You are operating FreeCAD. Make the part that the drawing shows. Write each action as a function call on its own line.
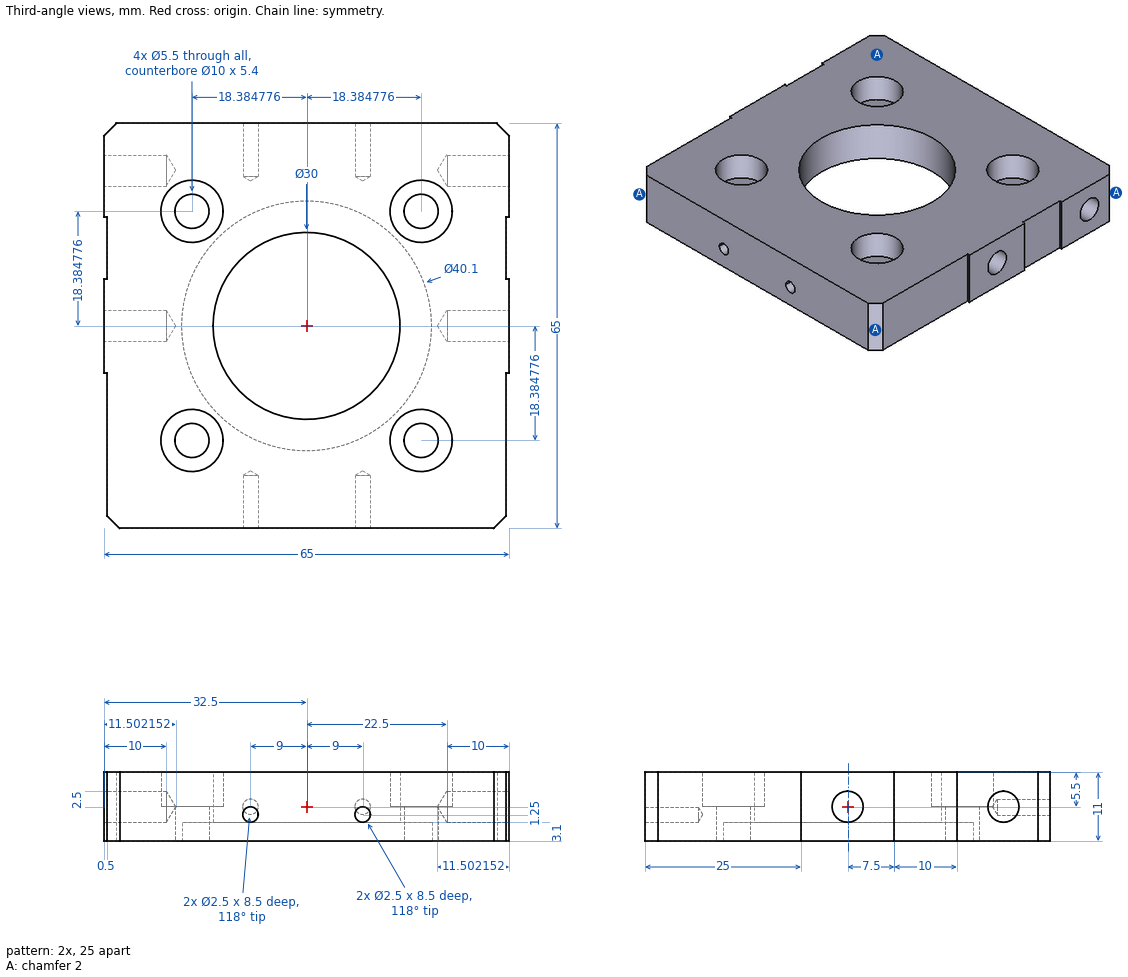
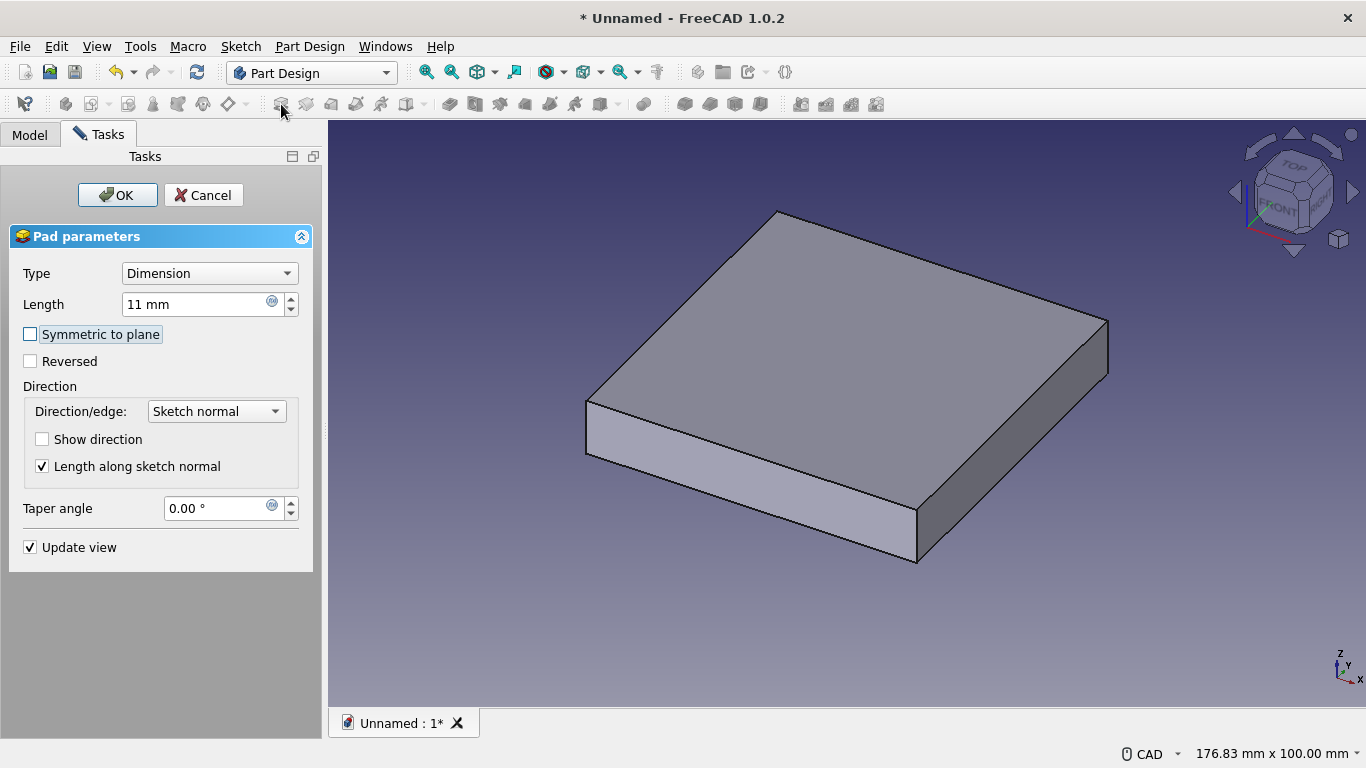
click(31, 334)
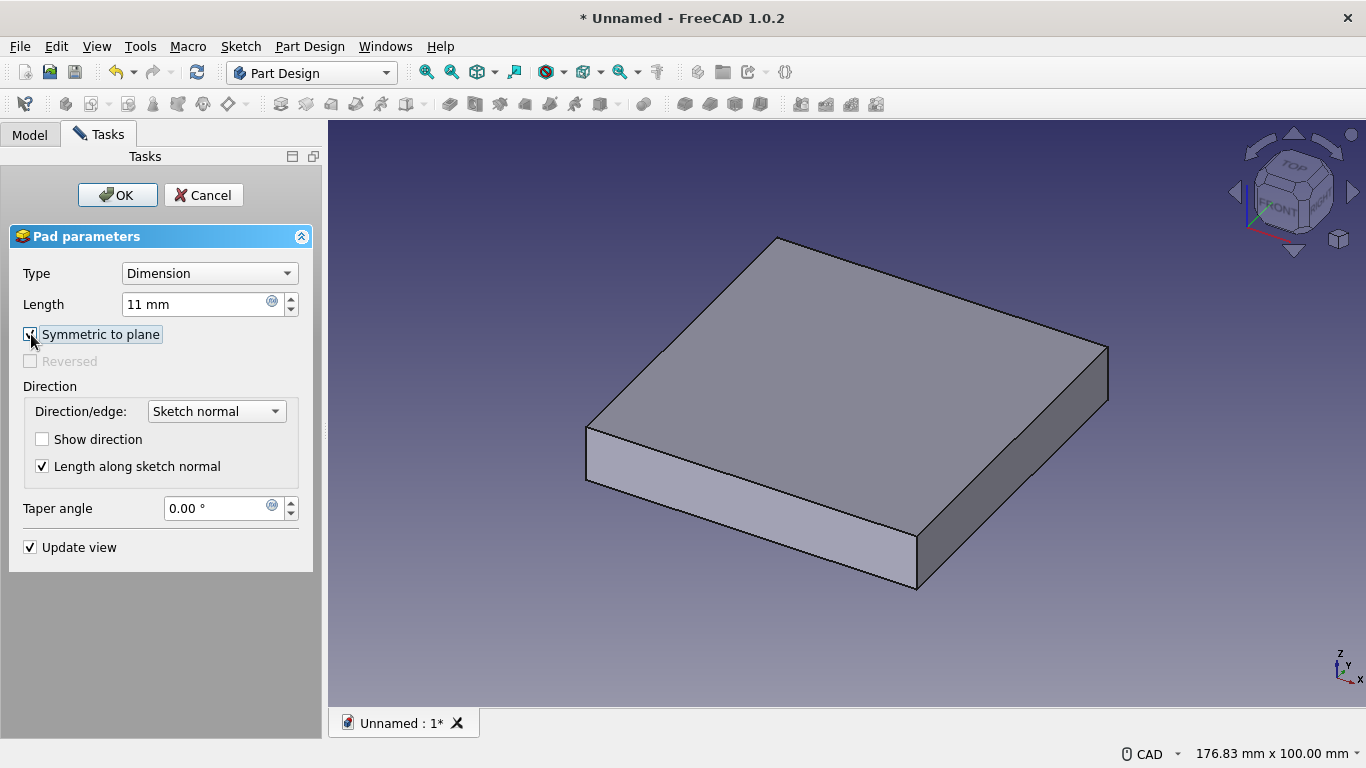
click(118, 195)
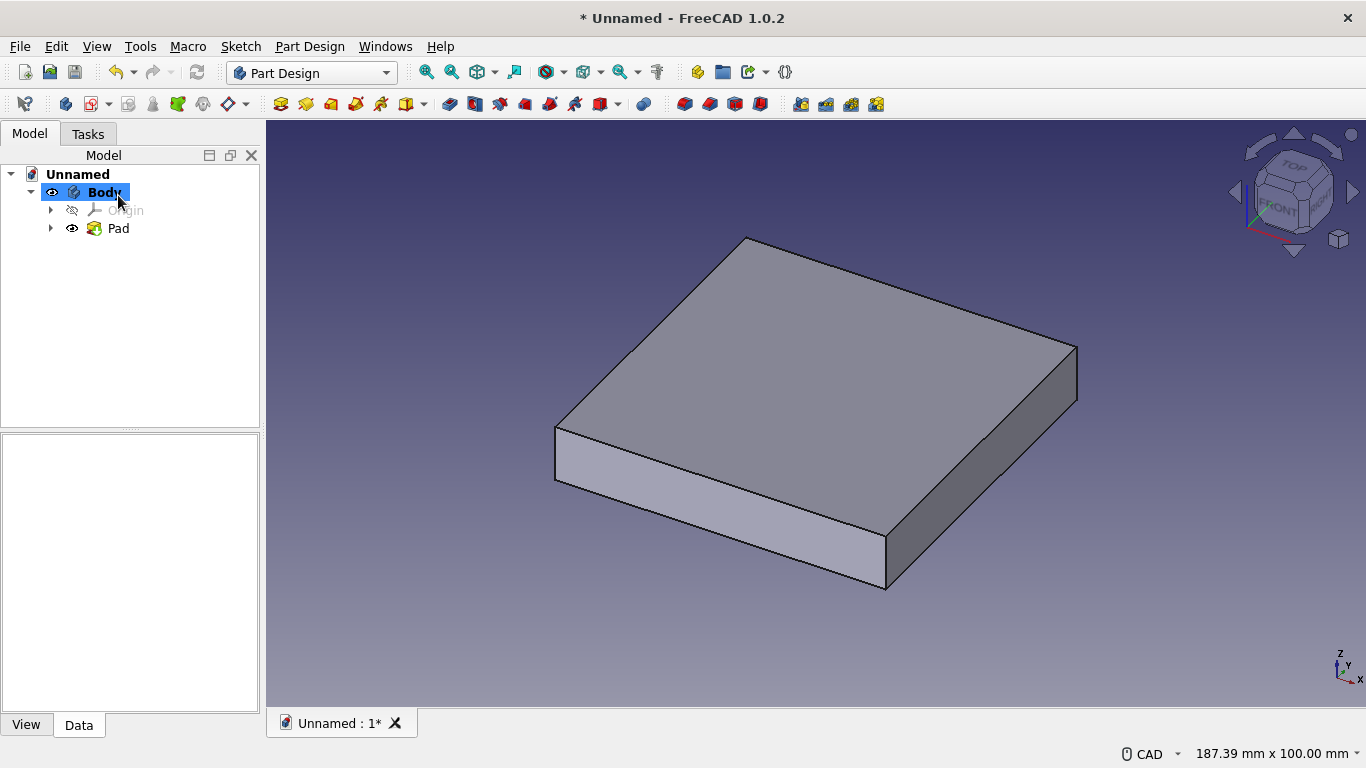
key(5)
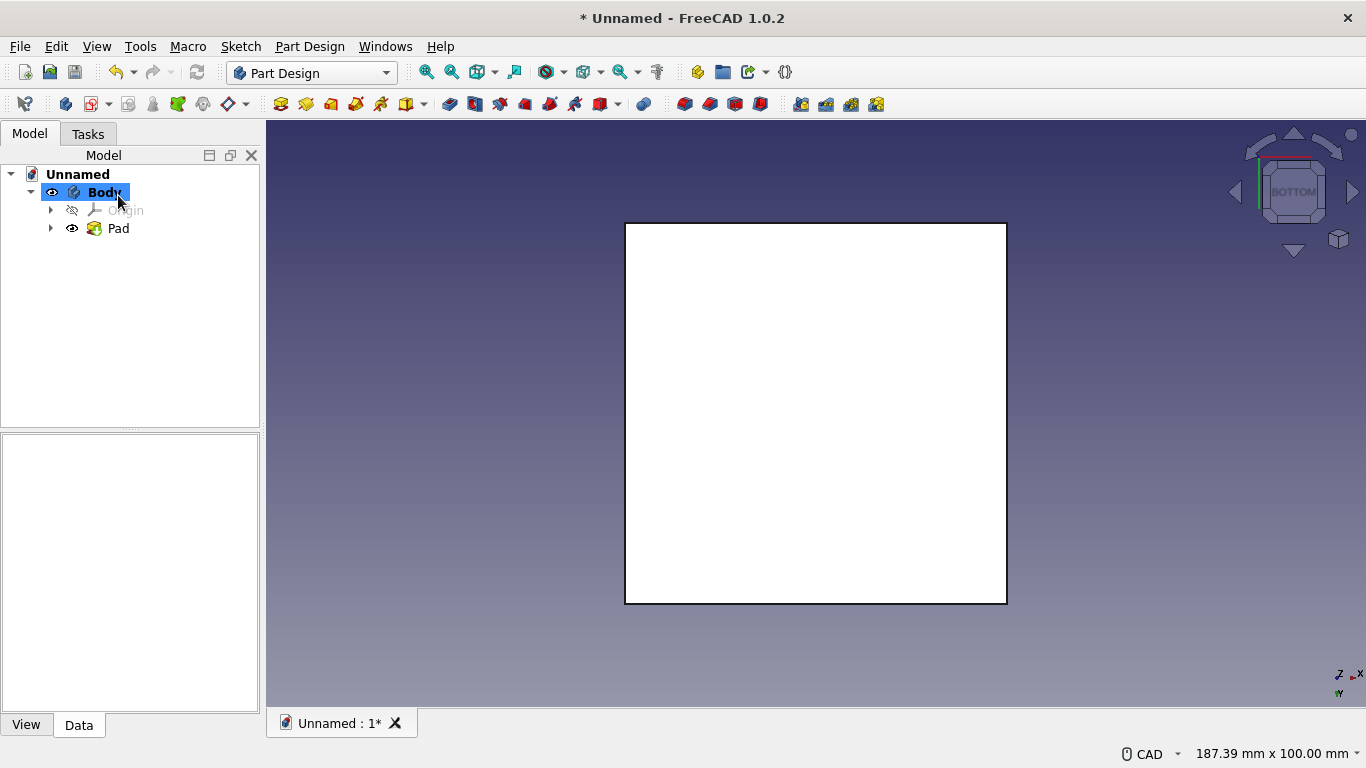
click(816, 412)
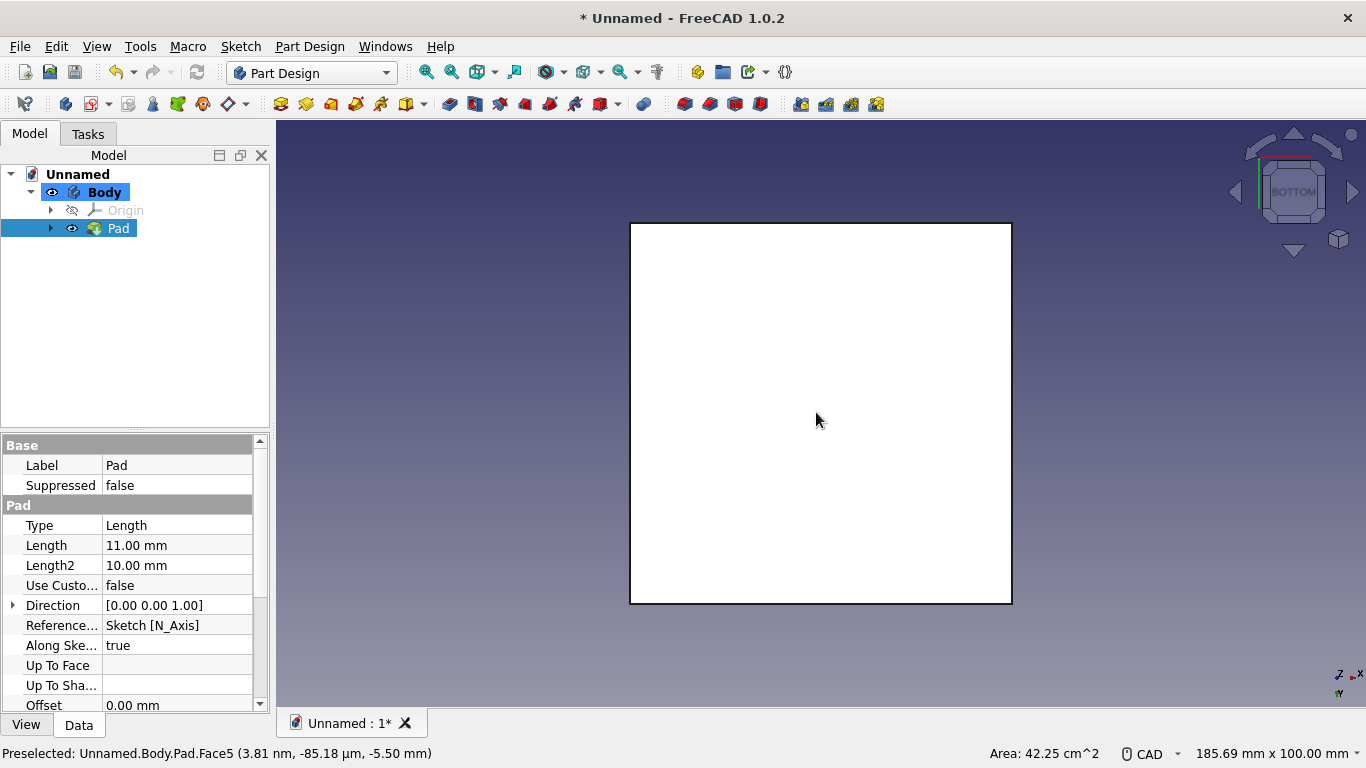
click(90, 104)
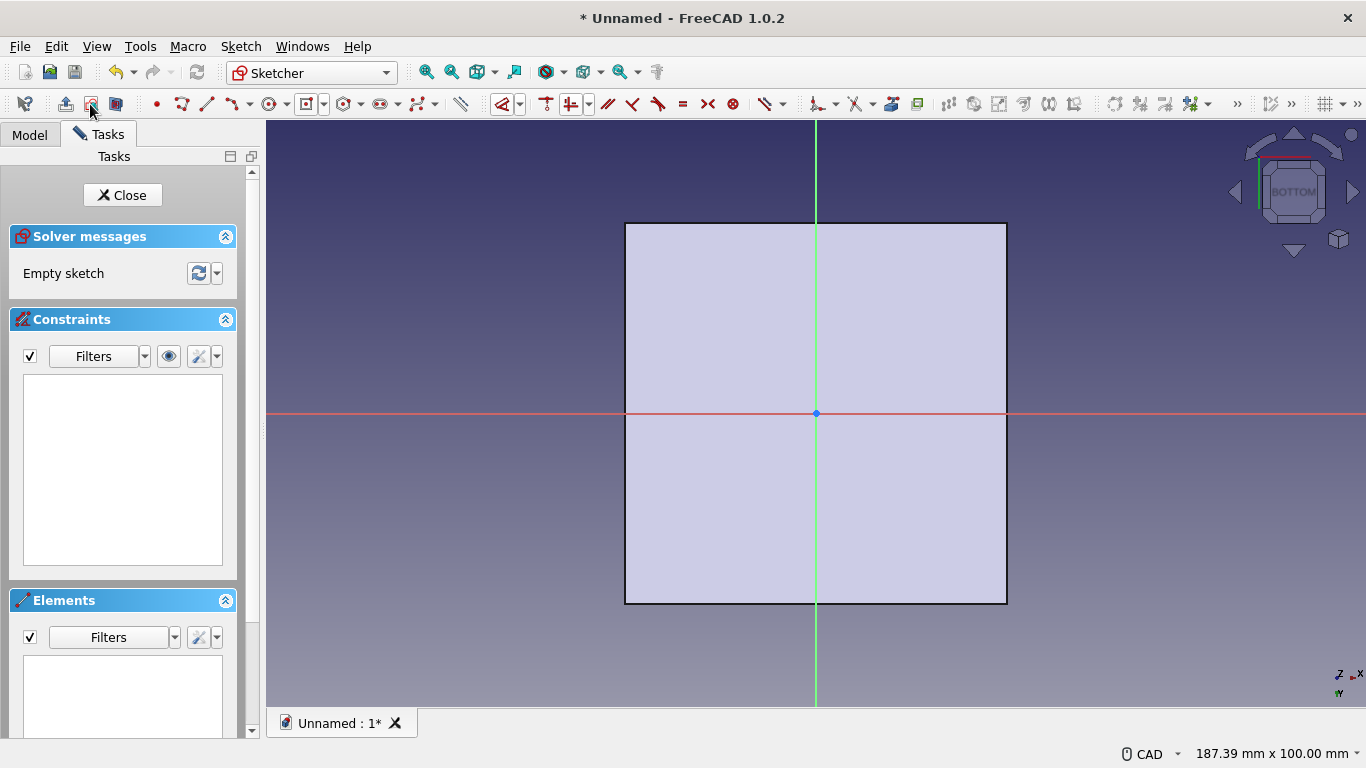
scroll(955, 413, up, 2)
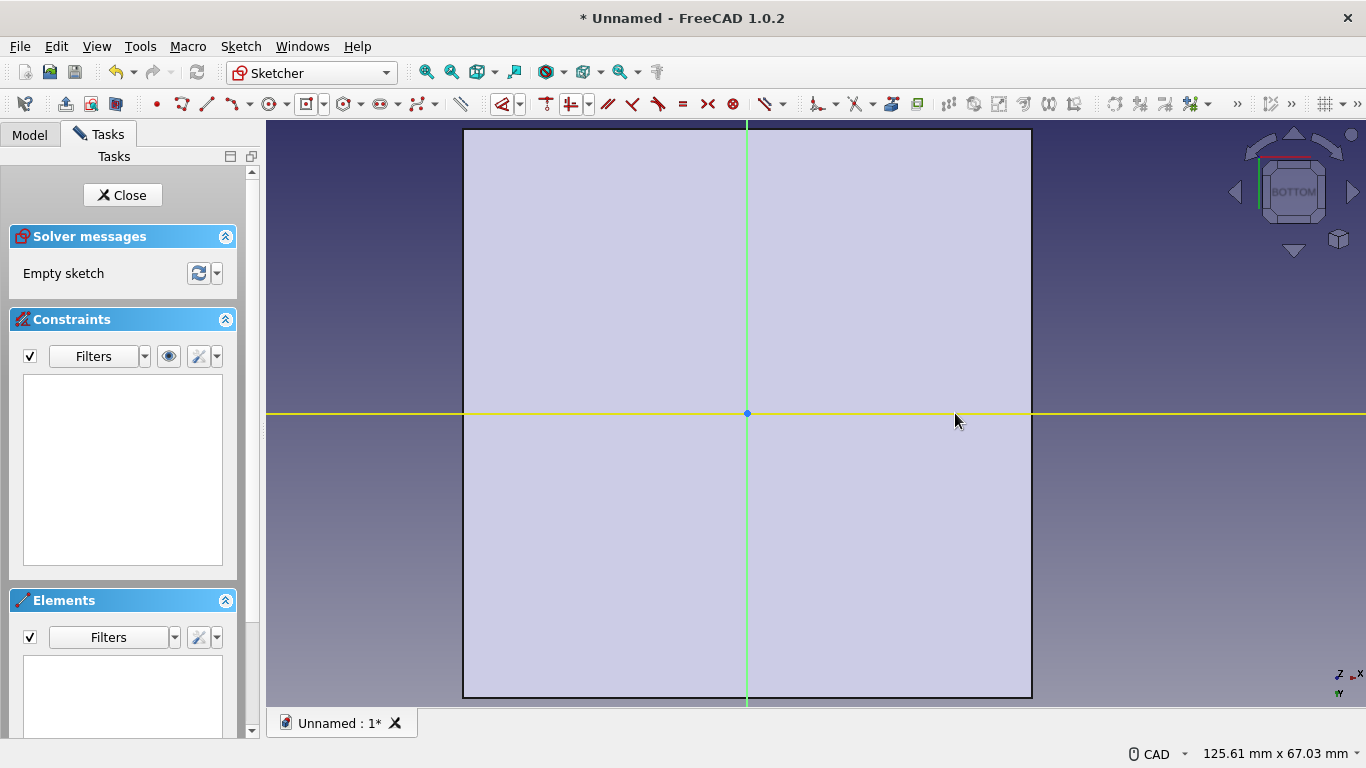
click(268, 104)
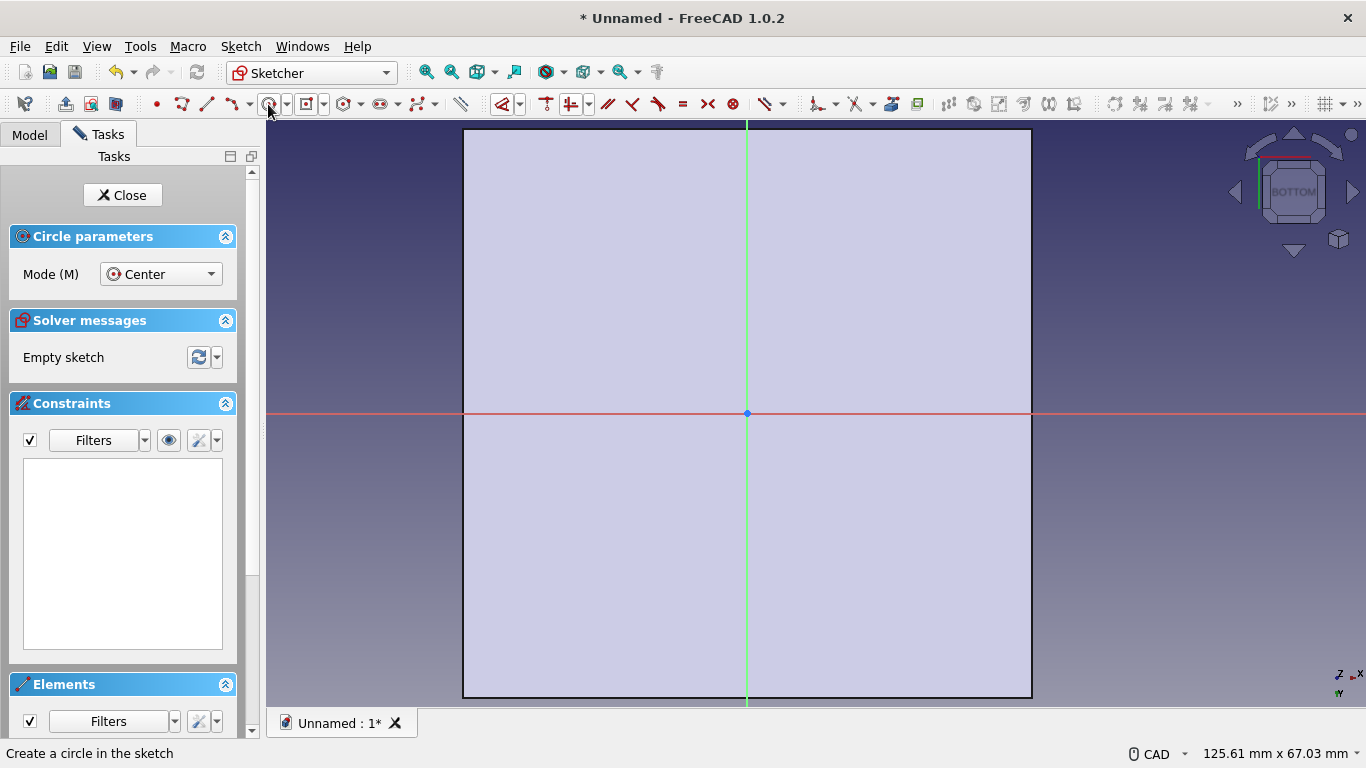
click(747, 414)
click(871, 289)
key(Escape)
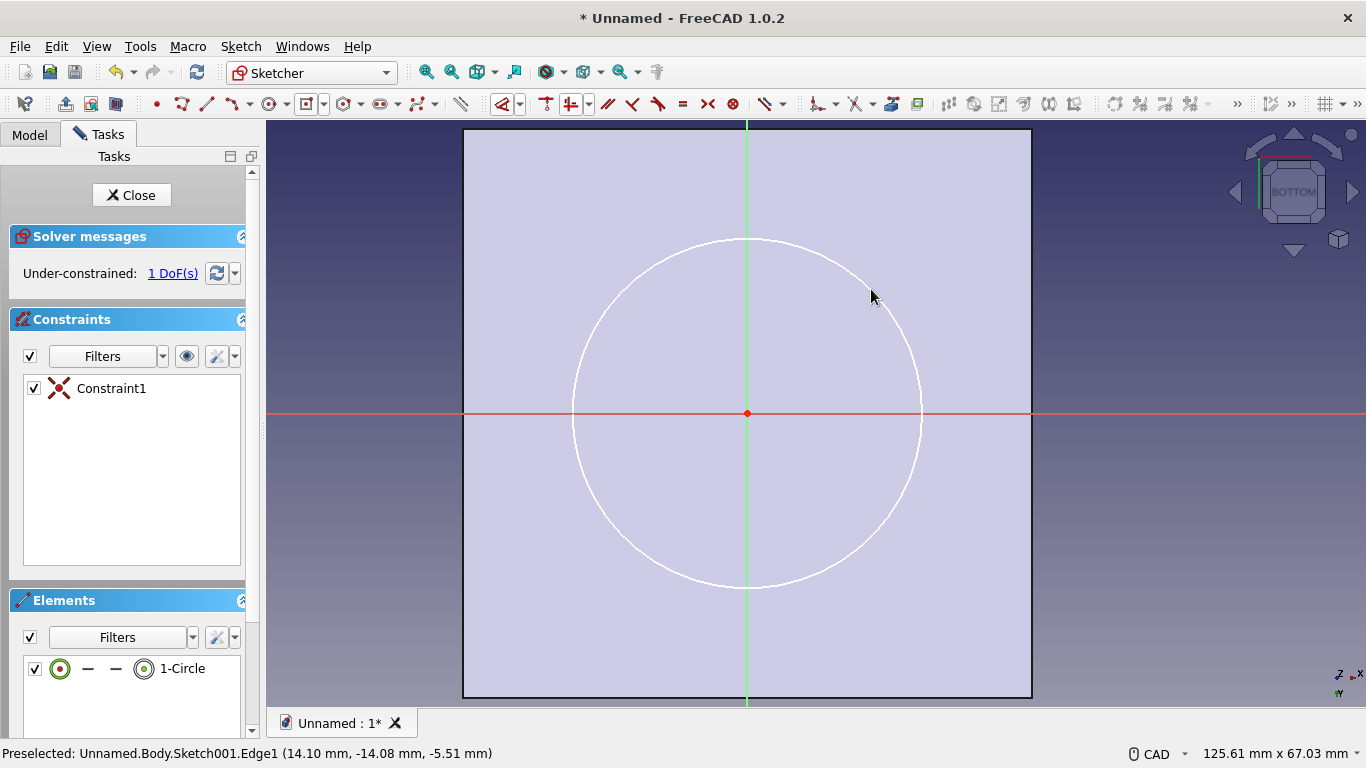
click(871, 290)